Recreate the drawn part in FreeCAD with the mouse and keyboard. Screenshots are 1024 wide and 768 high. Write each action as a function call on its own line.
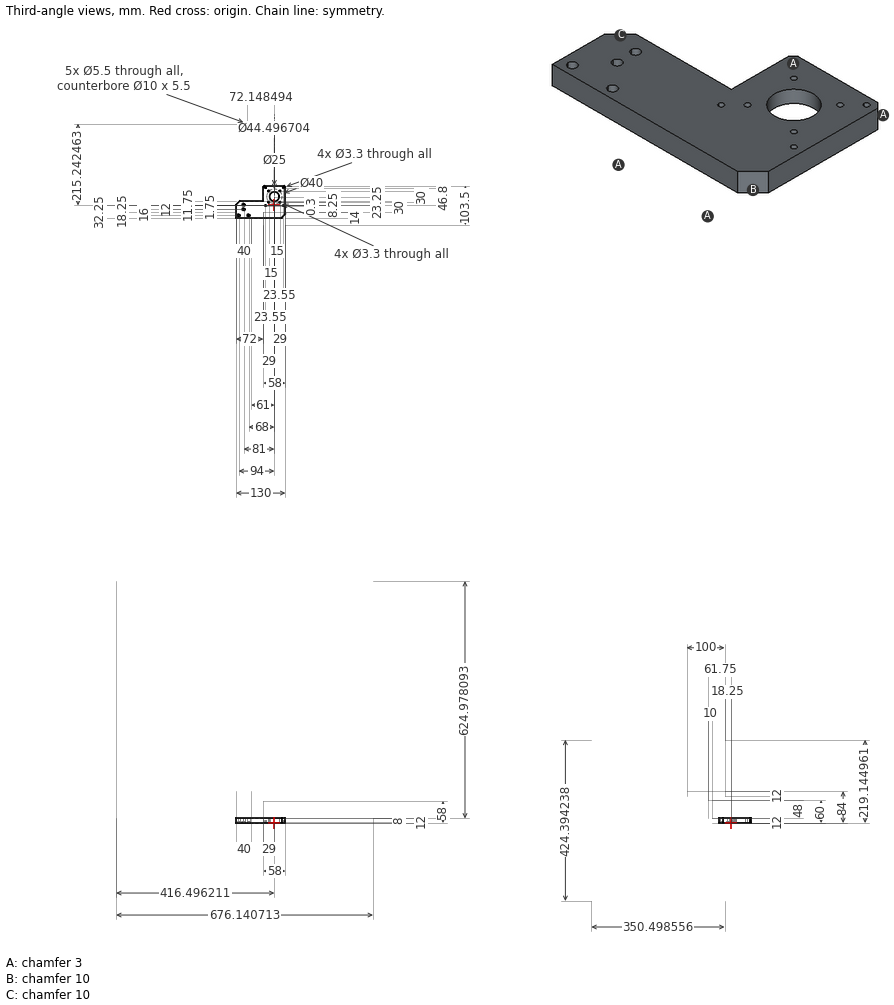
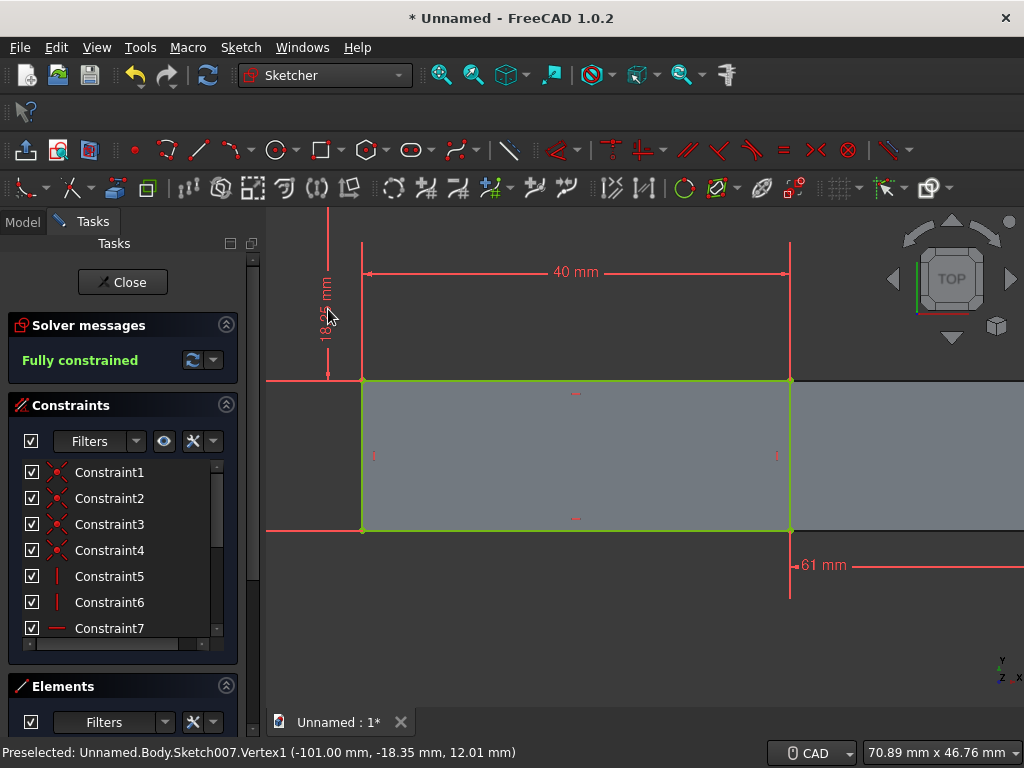
click(123, 282)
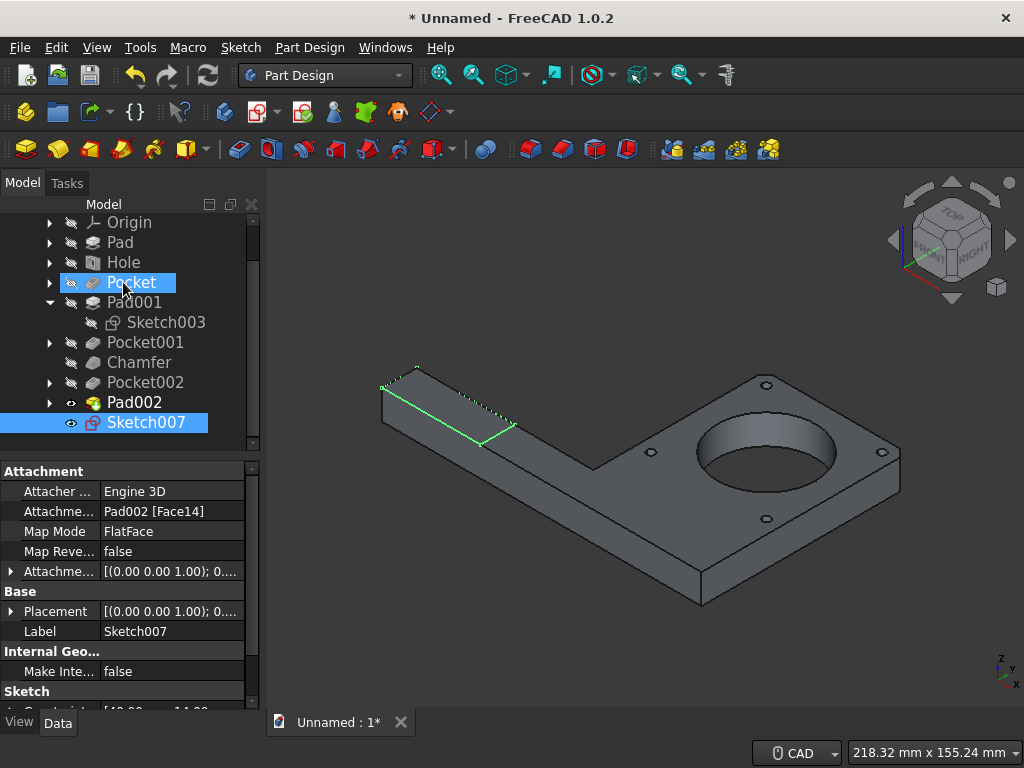
click(26, 150)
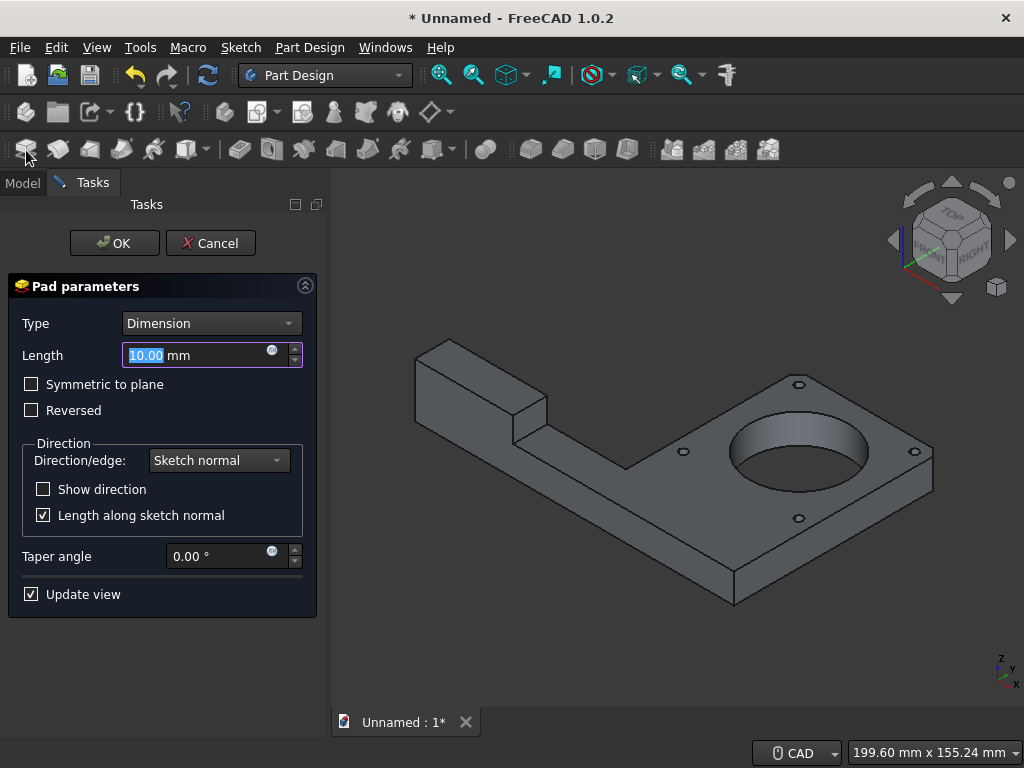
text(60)
key(Tab)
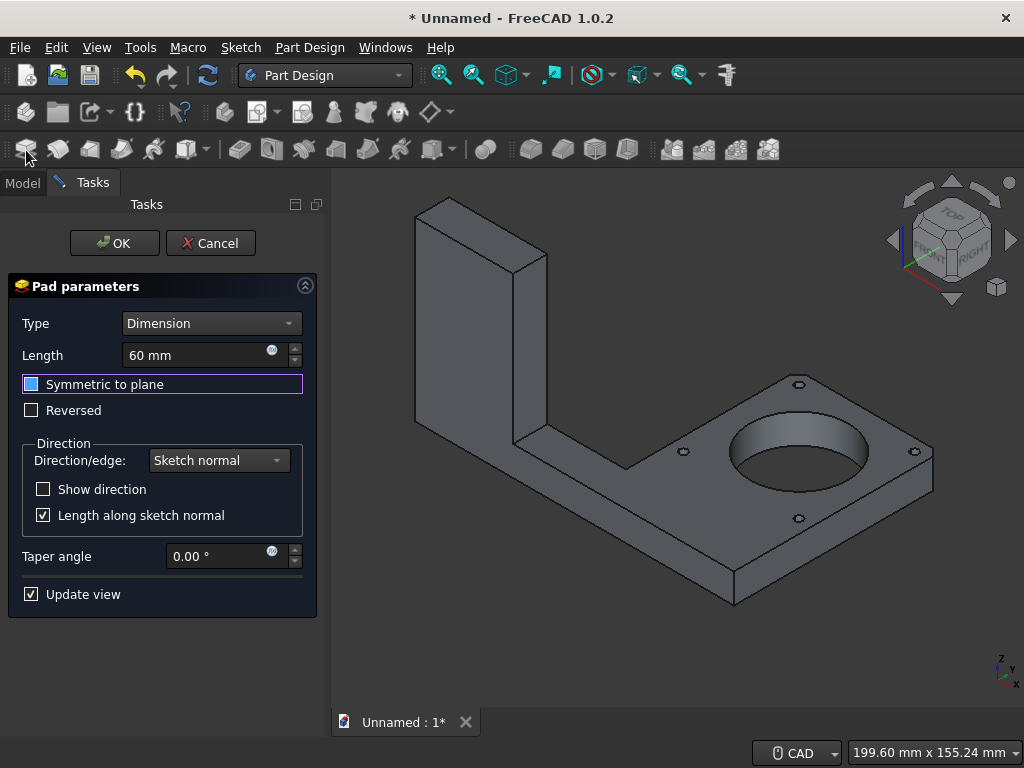
click(115, 243)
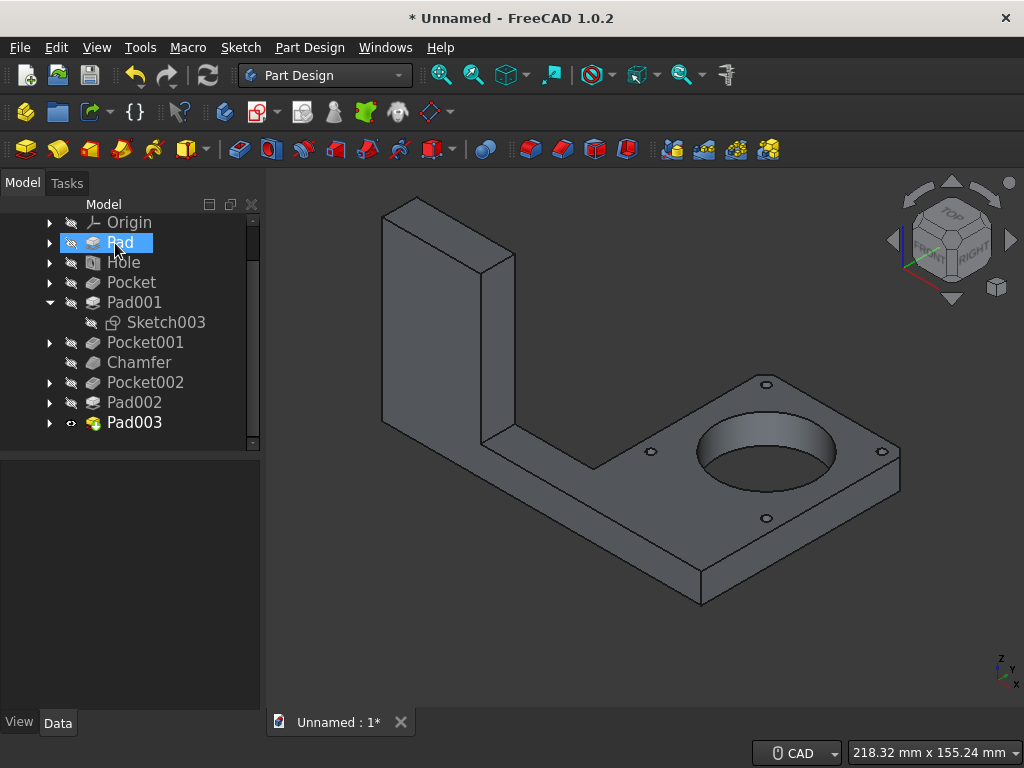
click(442, 76)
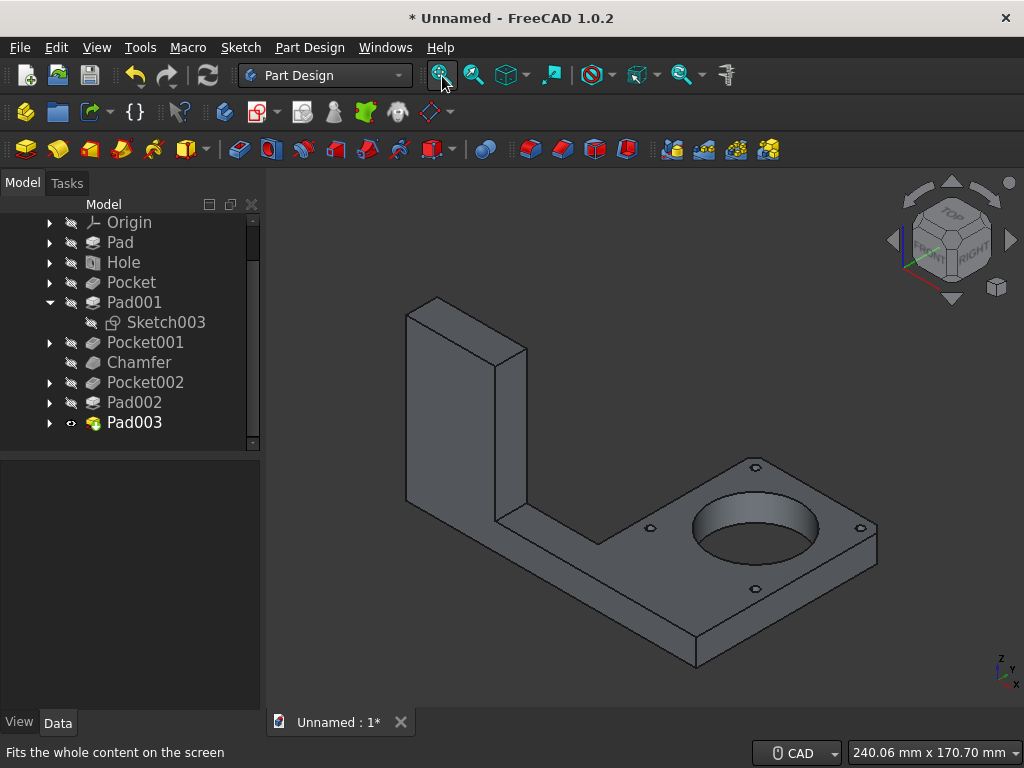
click(511, 390)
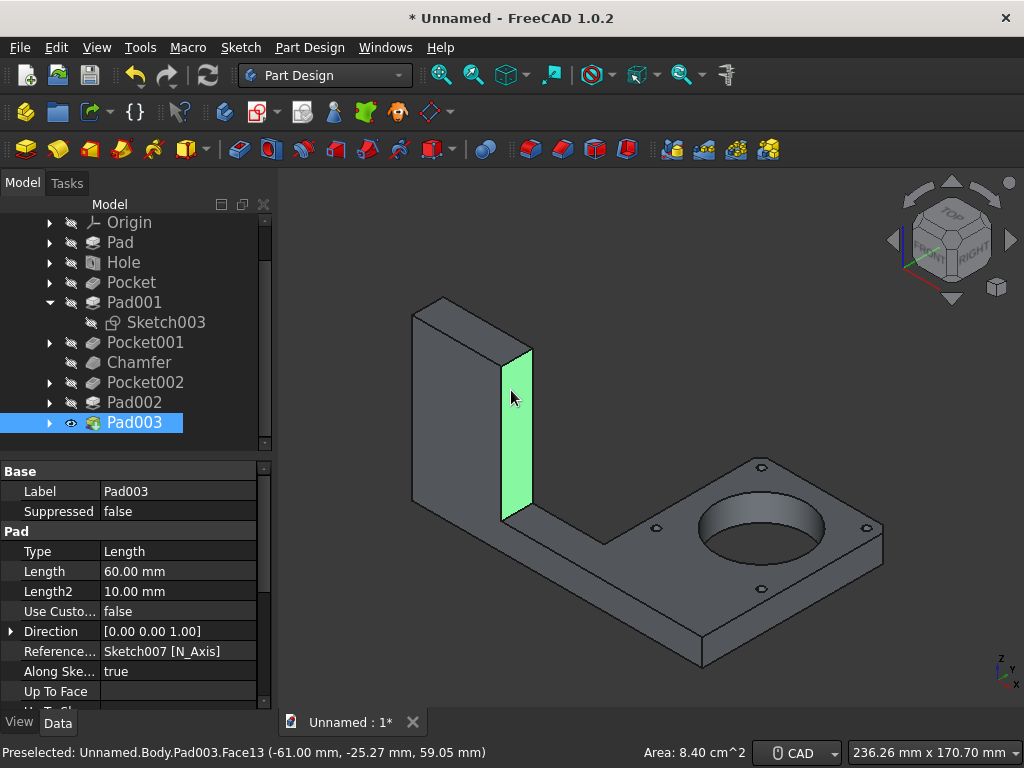
click(258, 112)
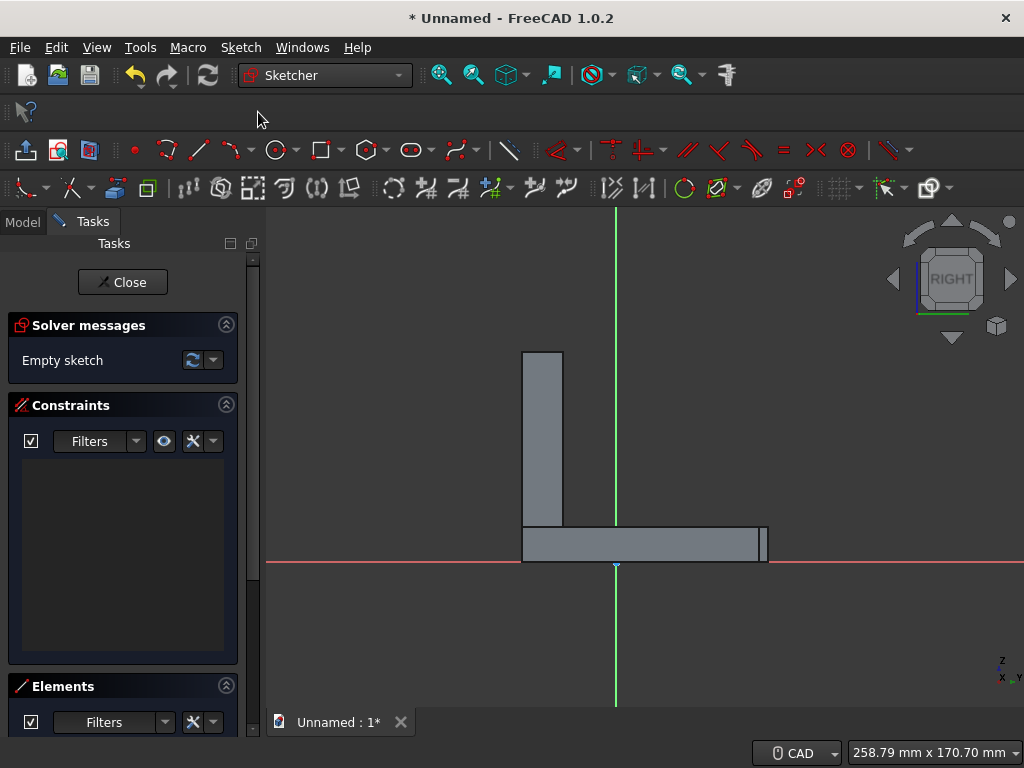
click(90, 150)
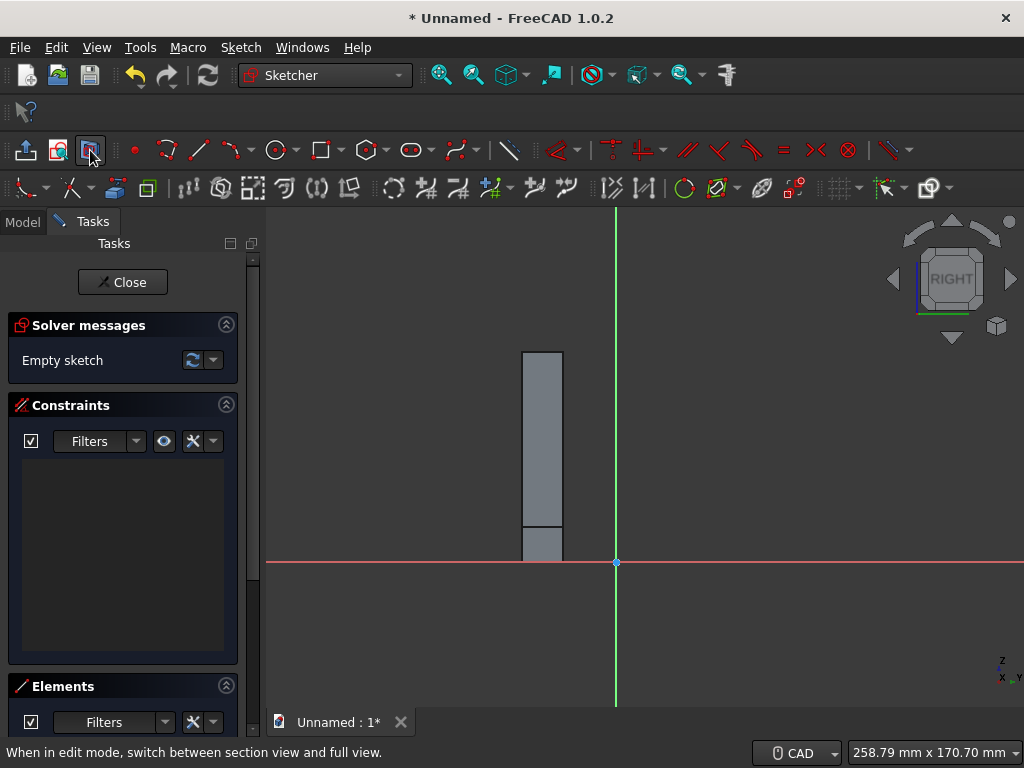
scroll(859, 536, down, 1)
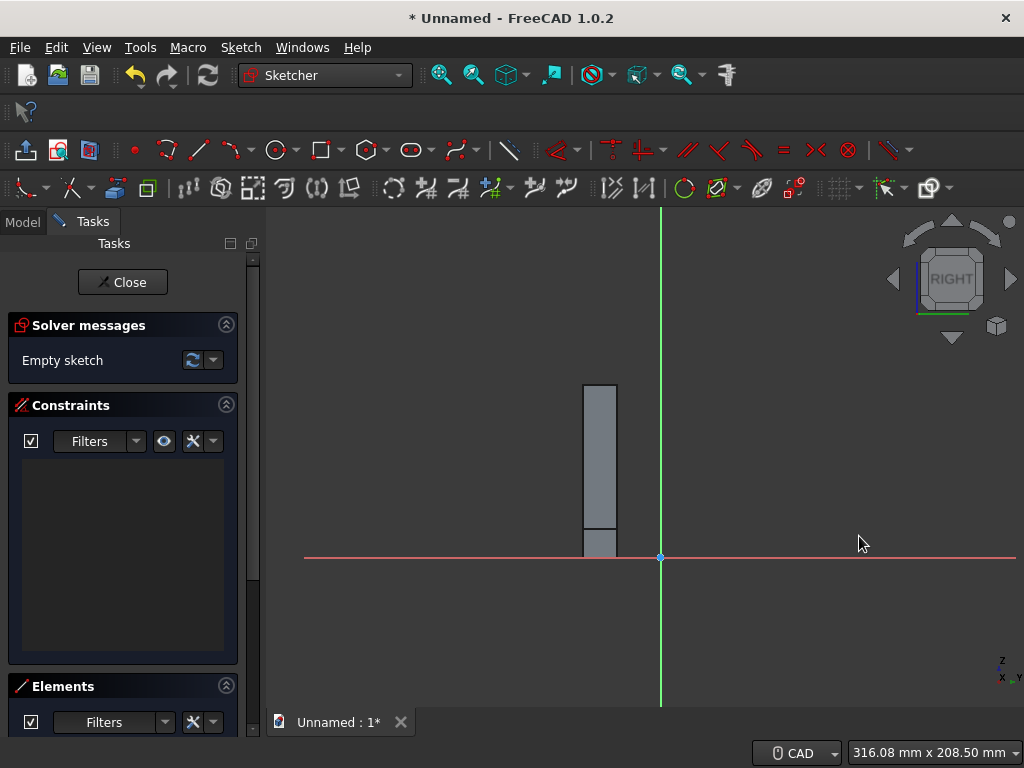
scroll(401, 457, up, 2)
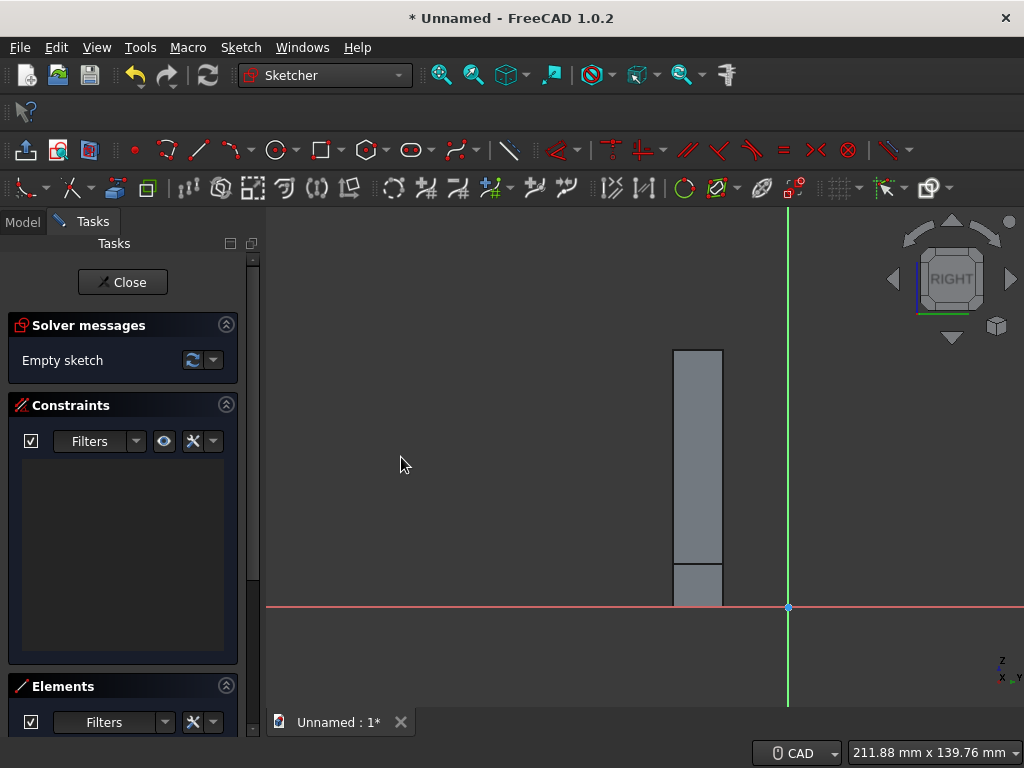
key(g)
key(r)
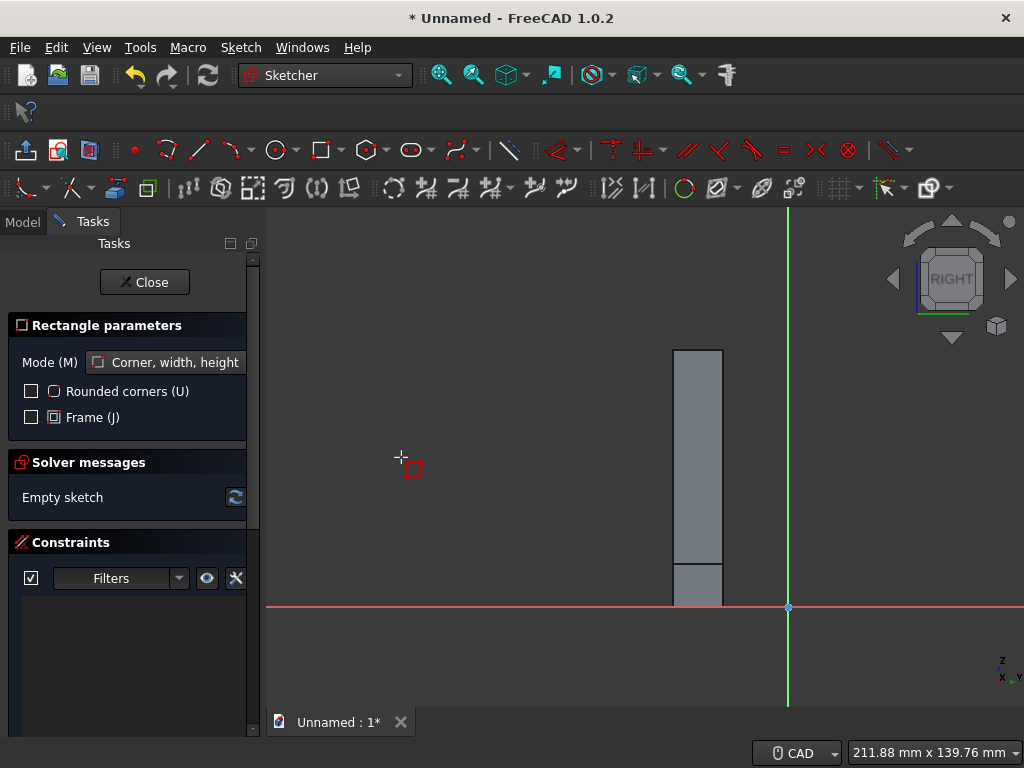
click(365, 307)
move(723, 350)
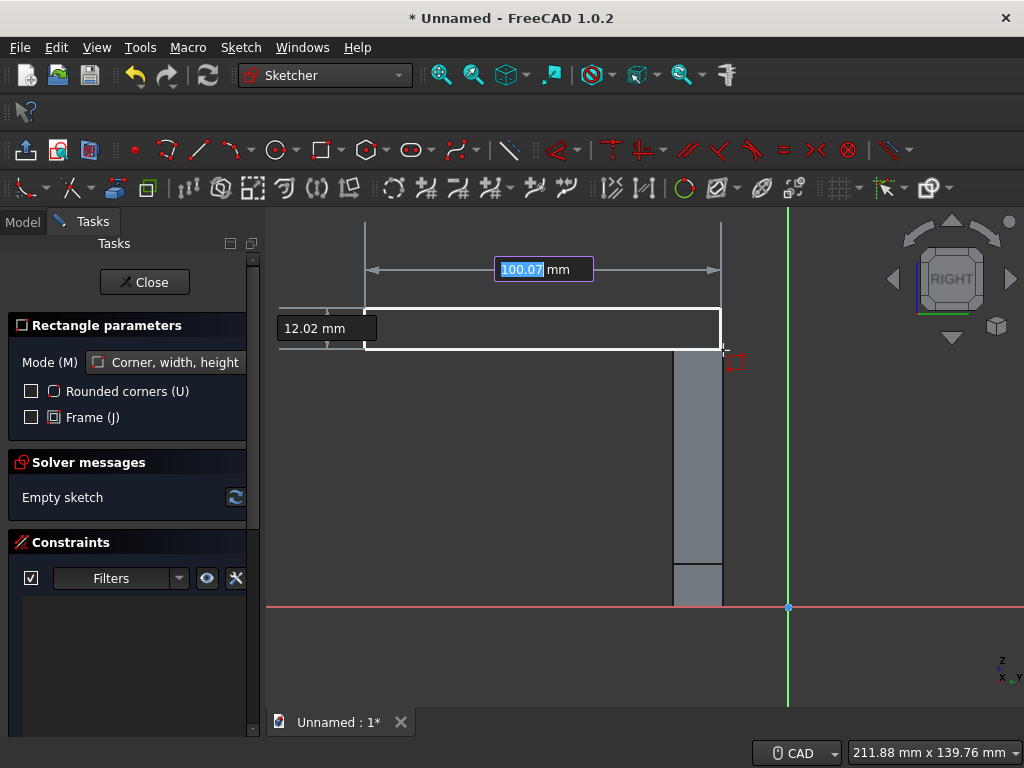
text(100)
key(Tab)
text(12)
key(Return)
key(Escape)